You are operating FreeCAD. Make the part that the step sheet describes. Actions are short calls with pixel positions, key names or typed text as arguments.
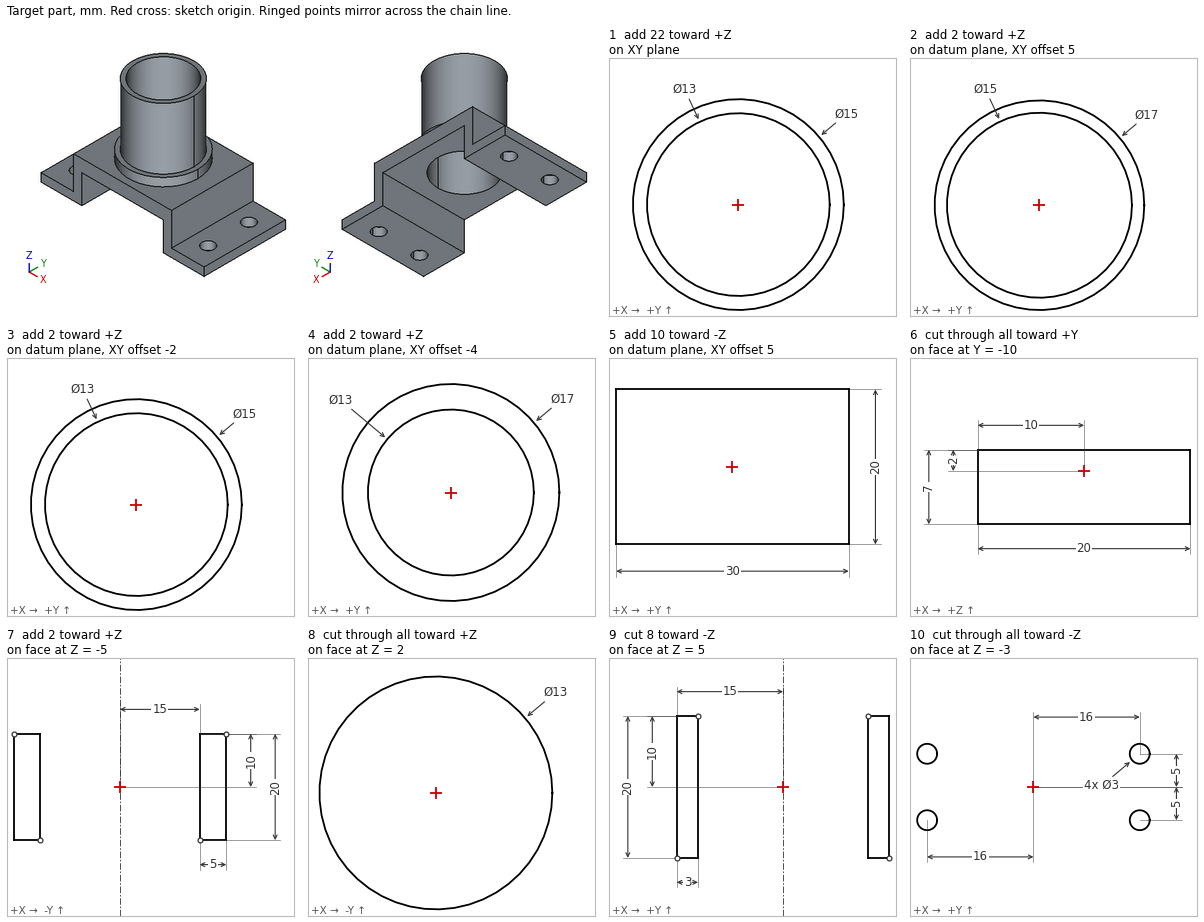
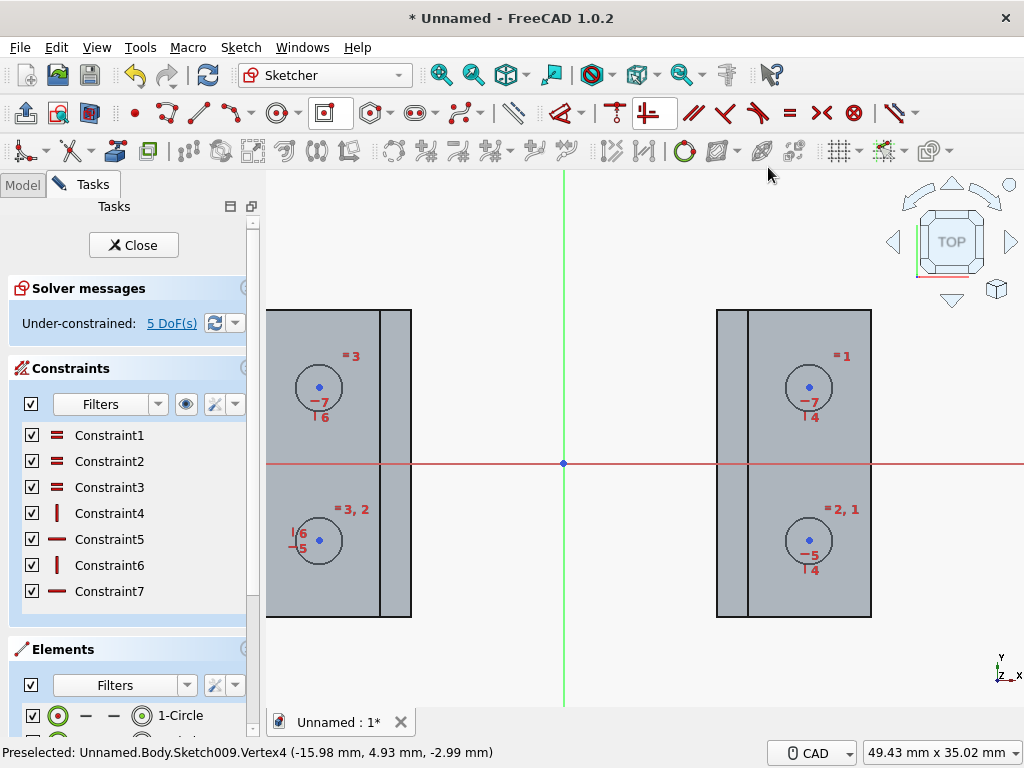
click(825, 371)
click(847, 348)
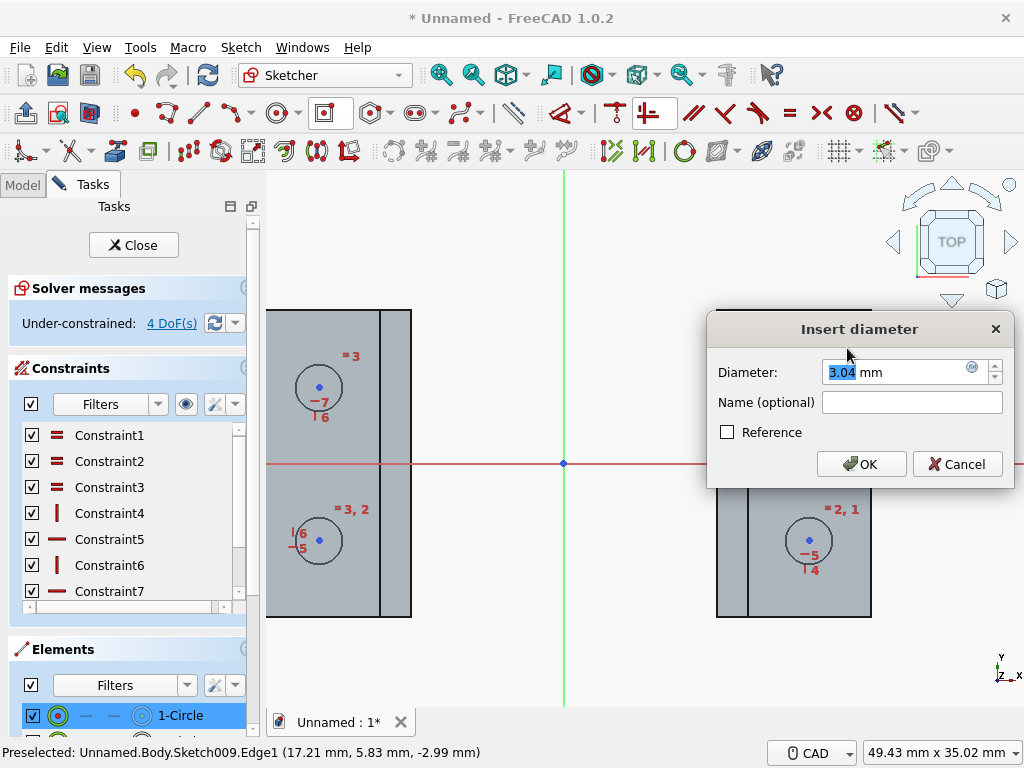
text(3)
key(Return)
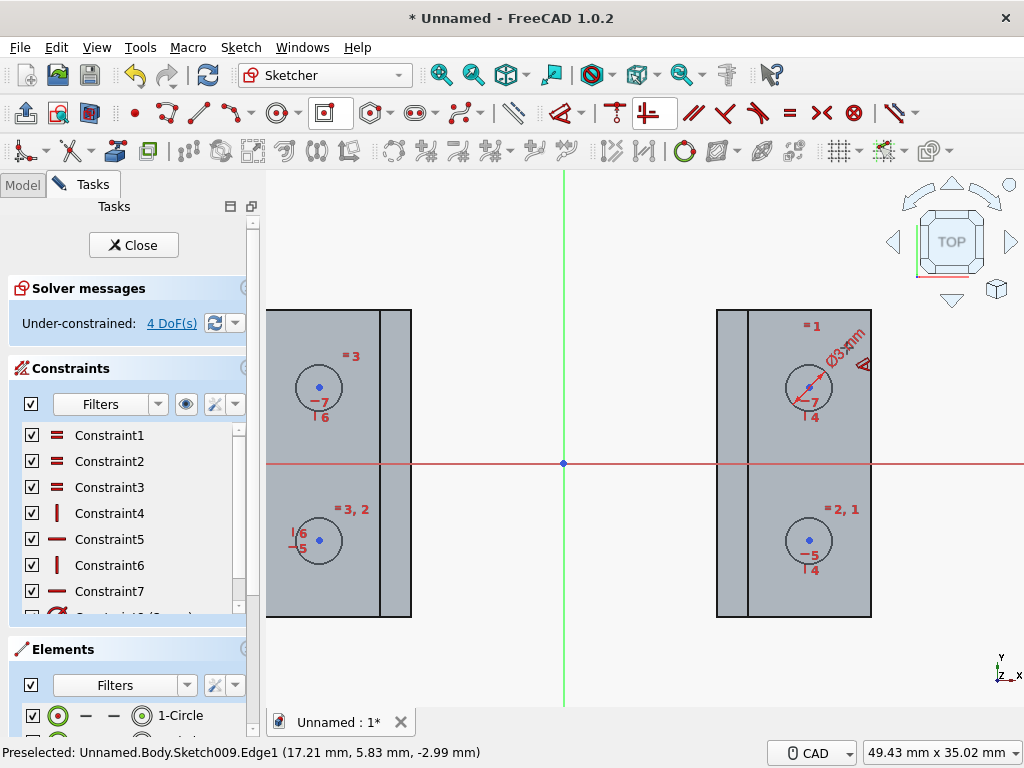
click(809, 388)
click(843, 426)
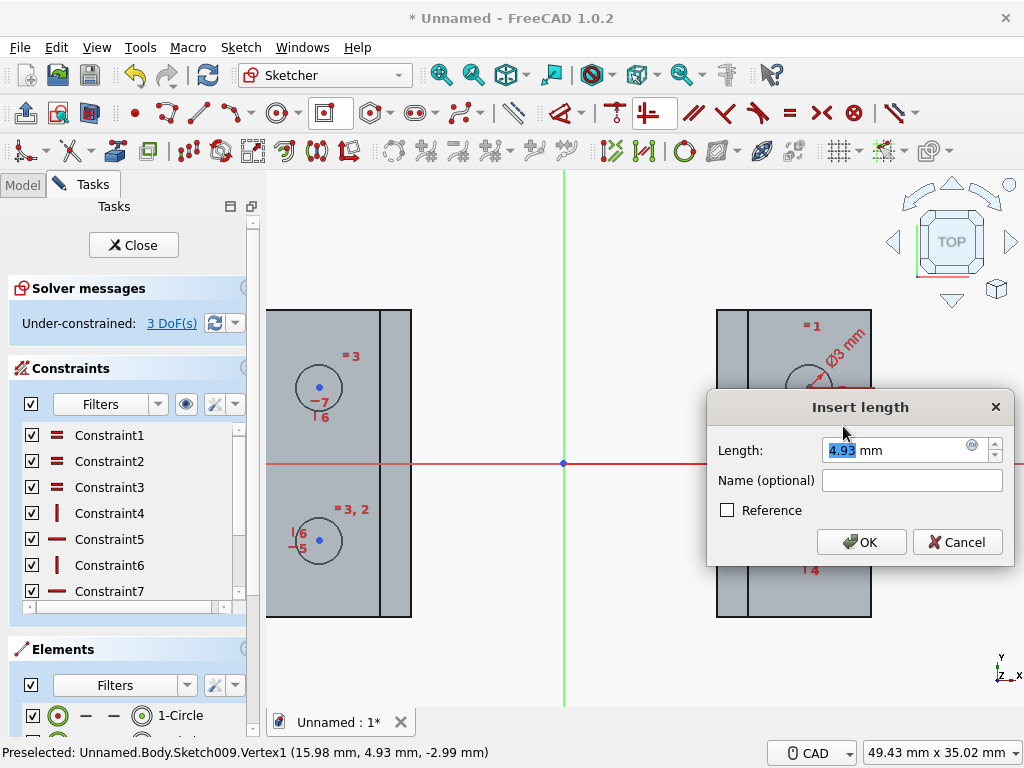
text(5)
key(Return)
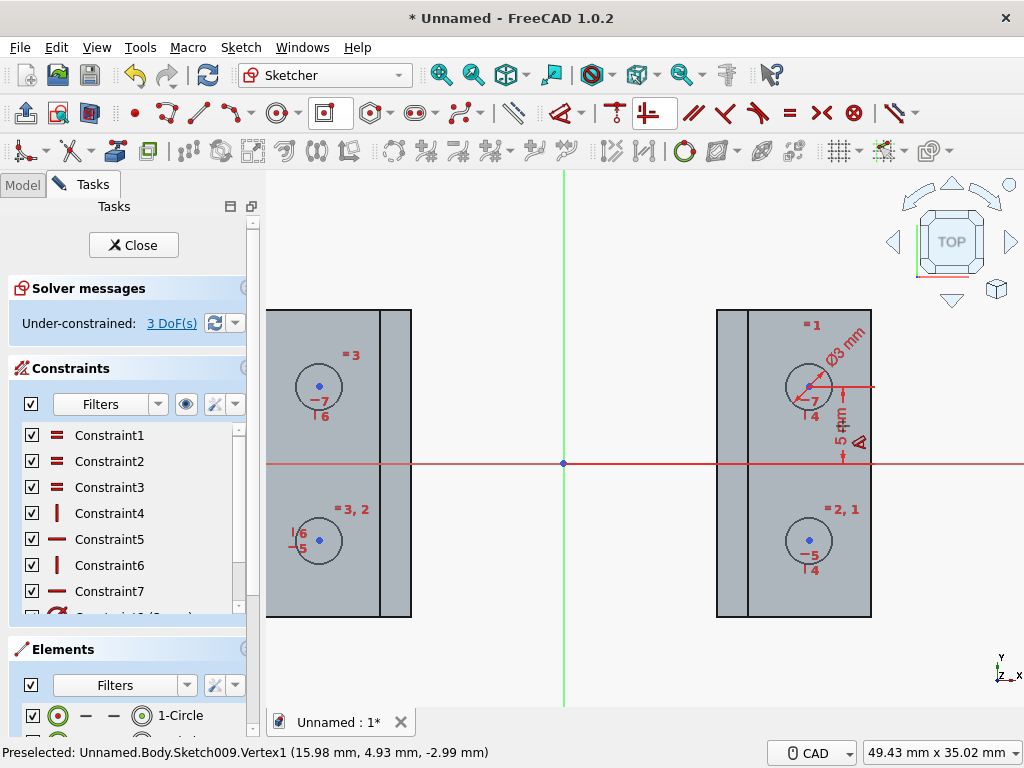
click(809, 541)
click(843, 502)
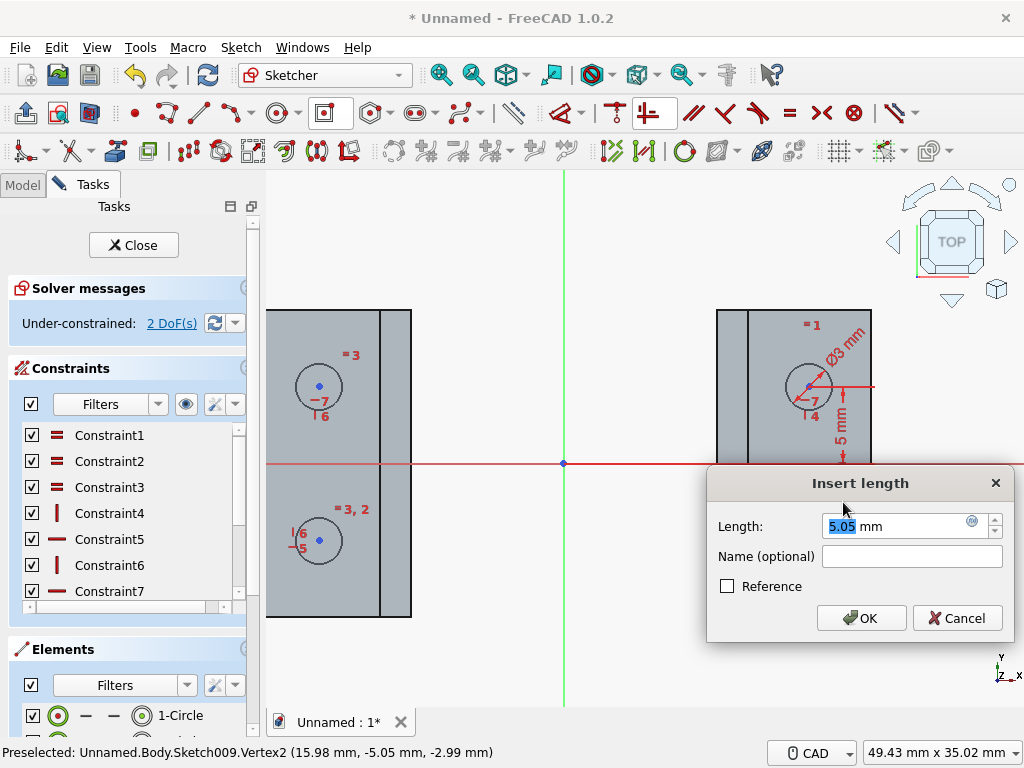
text(5)
key(Return)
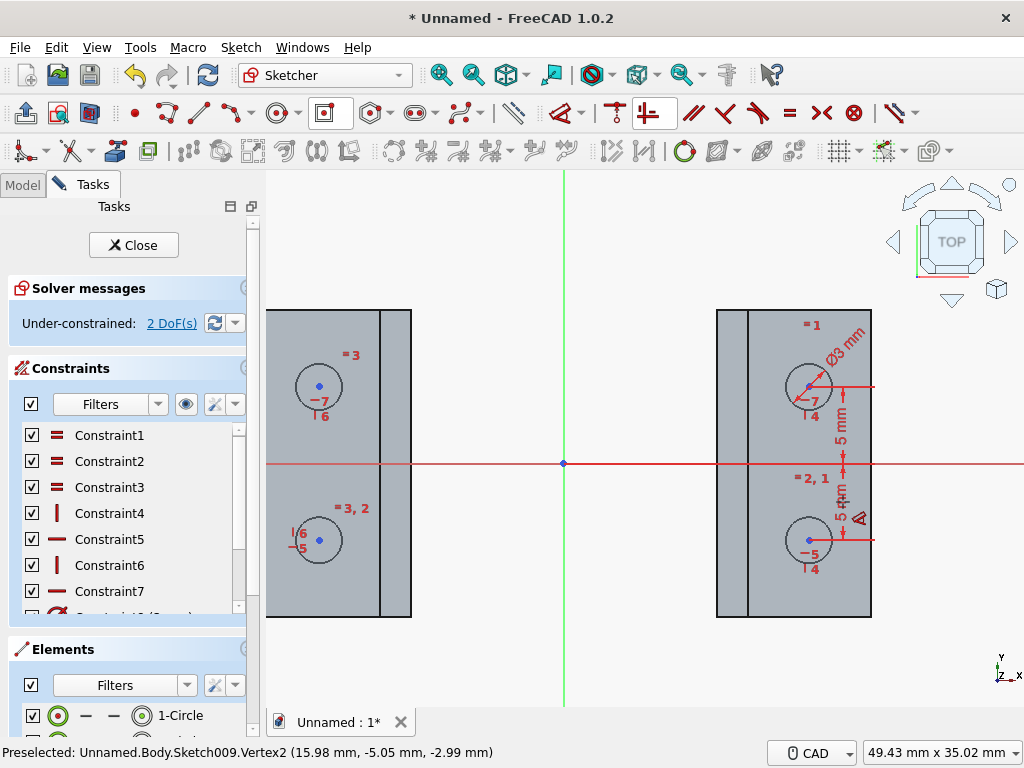
click(809, 387)
click(686, 353)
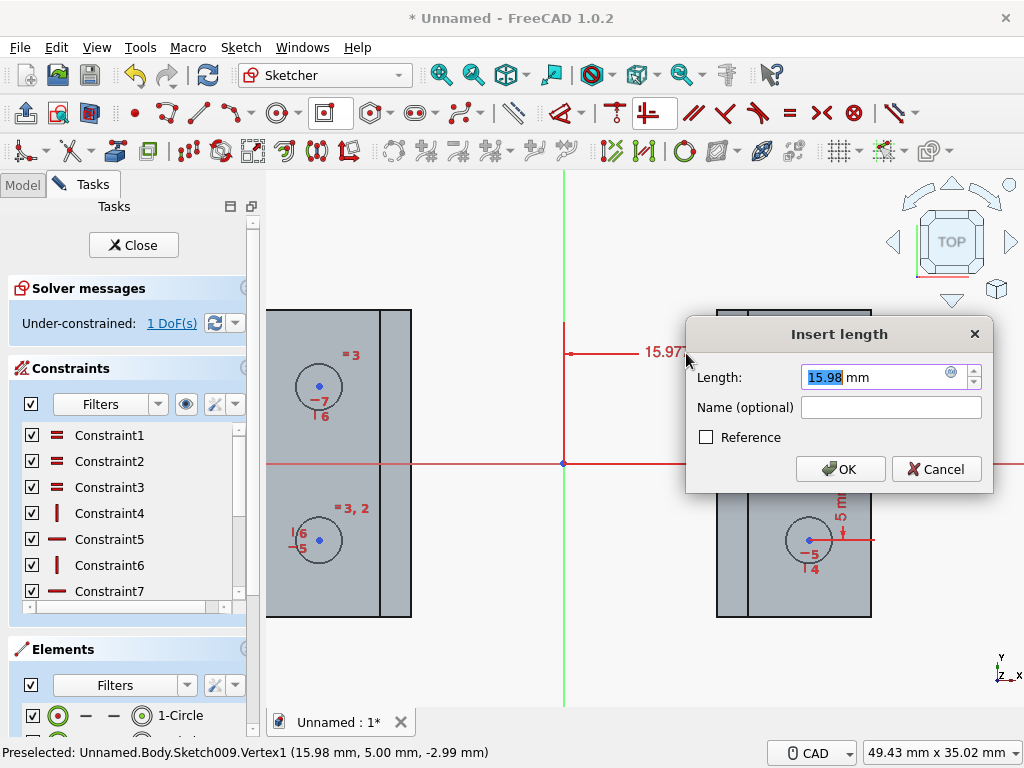
text(16)
key(Return)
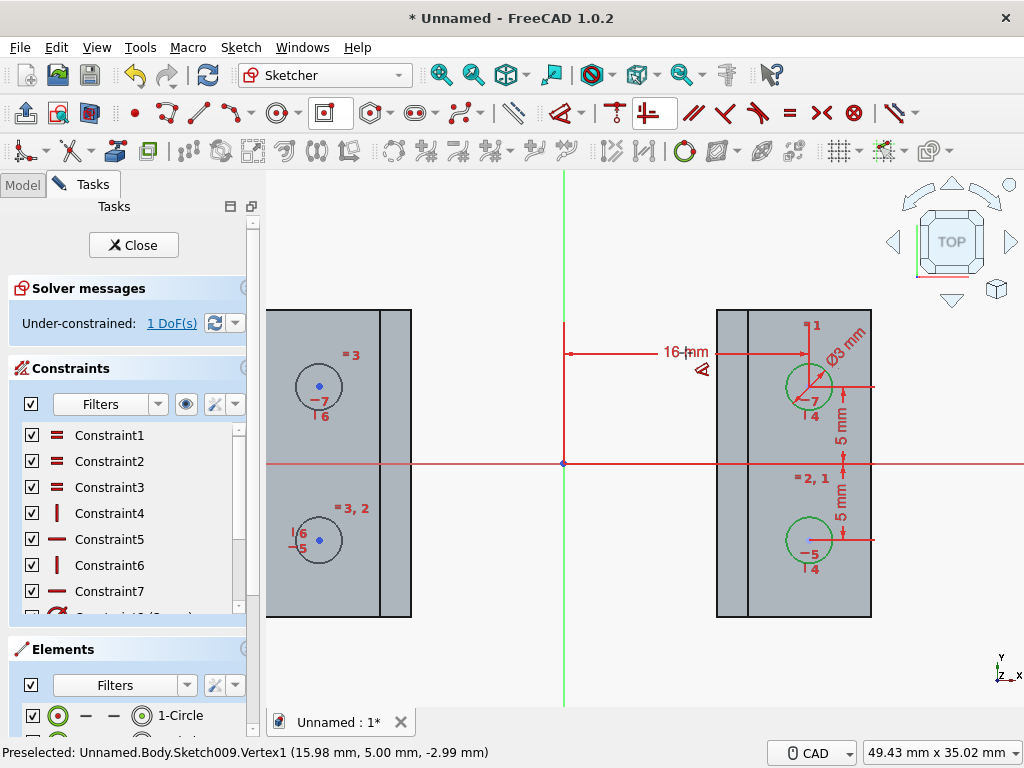
click(319, 540)
click(441, 574)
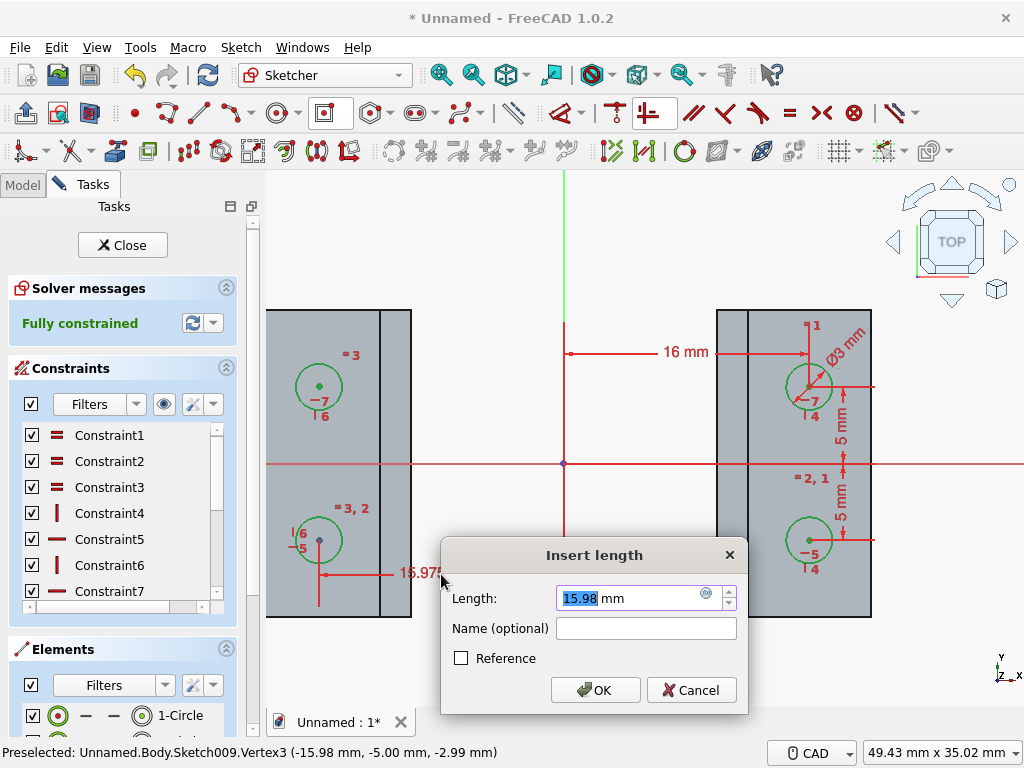
text(16)
key(Return)
key(Escape)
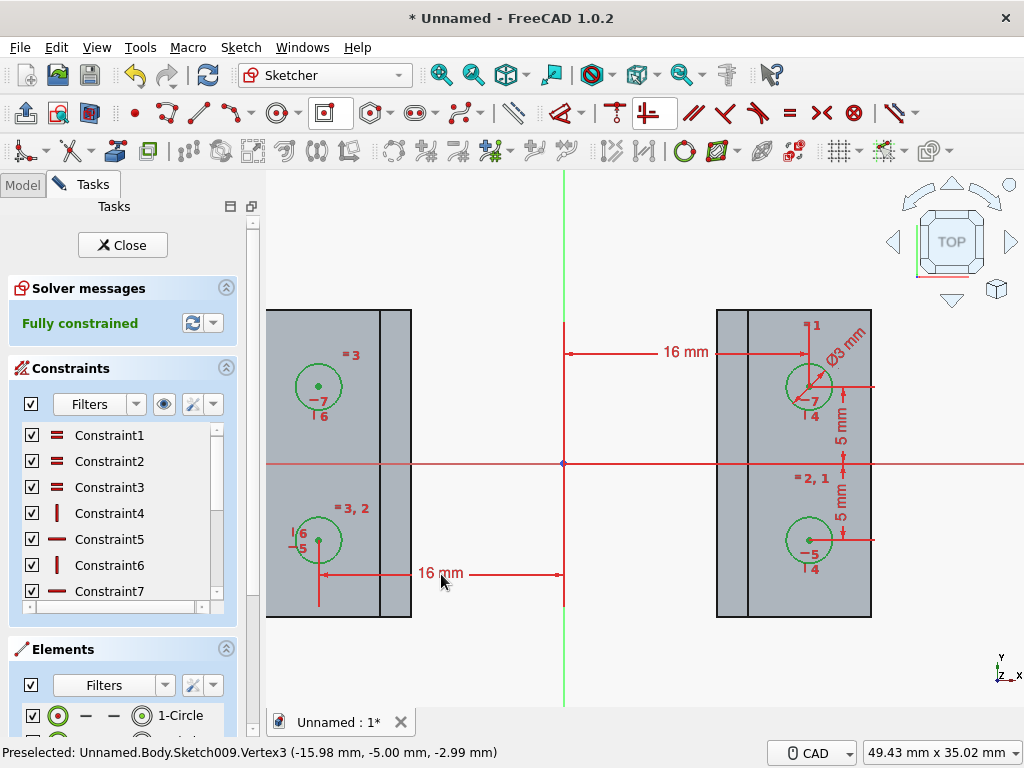
click(123, 245)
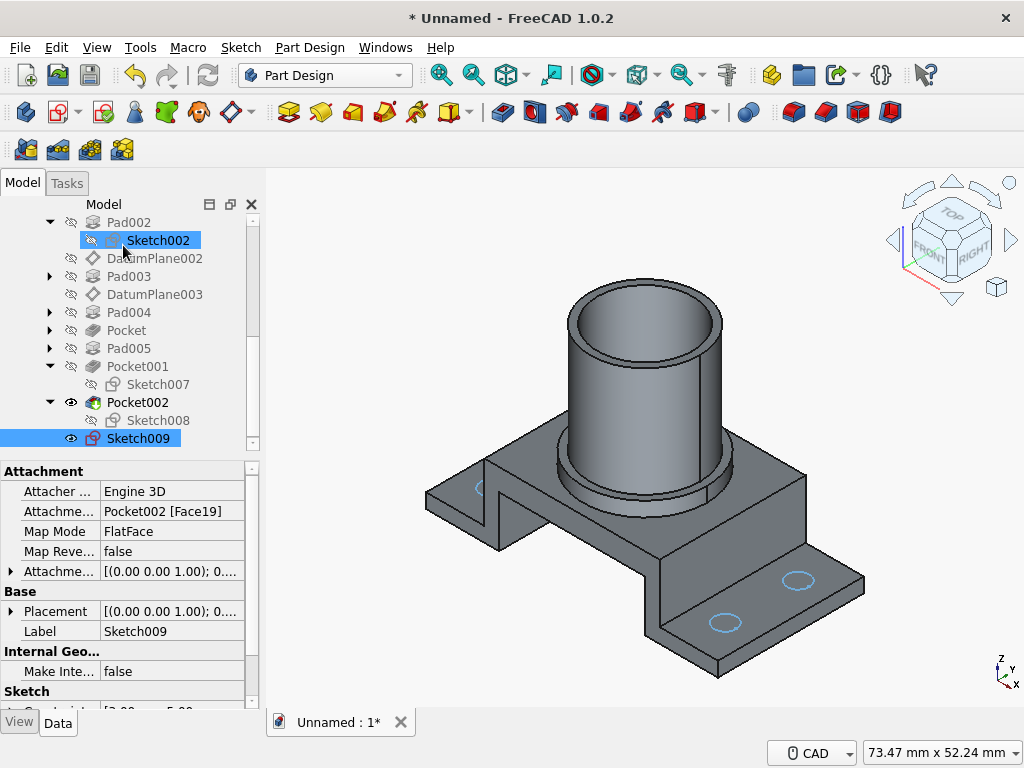
click(504, 112)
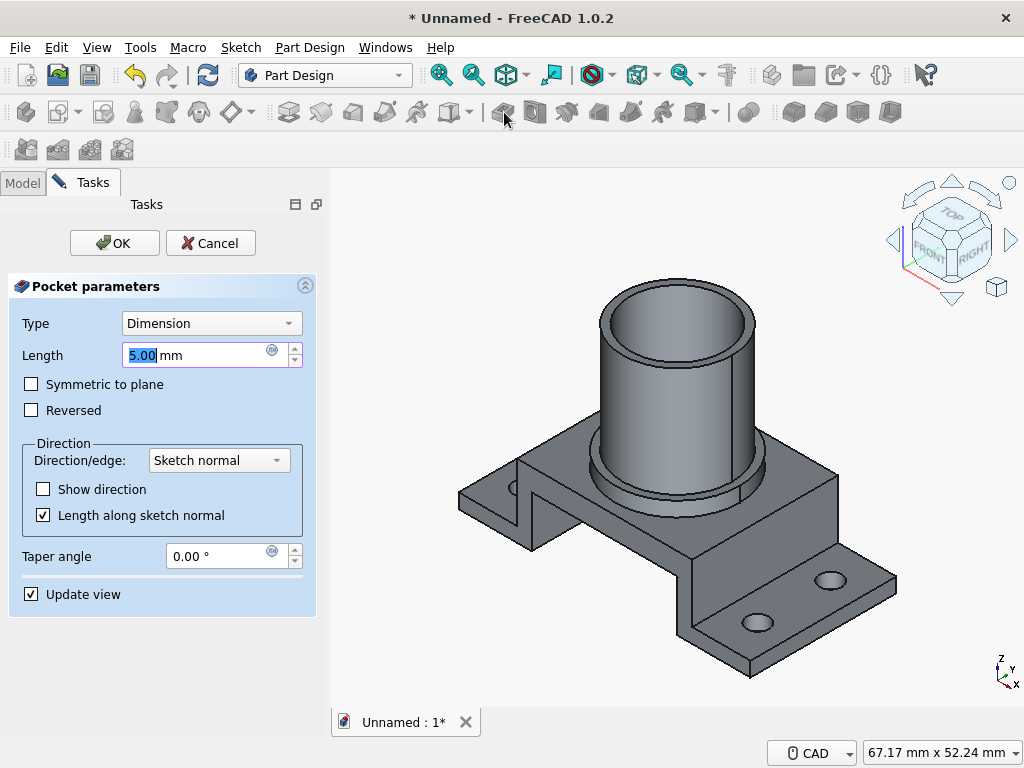
click(212, 324)